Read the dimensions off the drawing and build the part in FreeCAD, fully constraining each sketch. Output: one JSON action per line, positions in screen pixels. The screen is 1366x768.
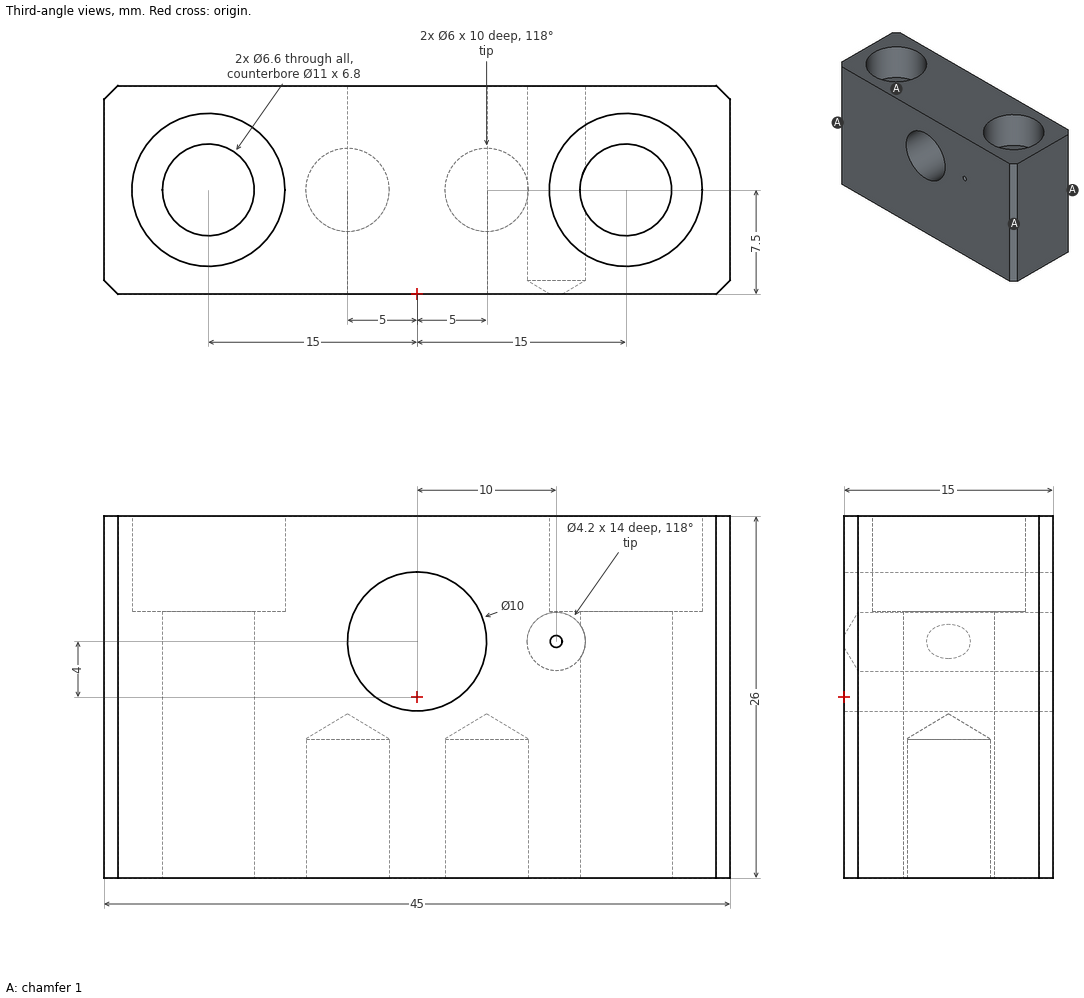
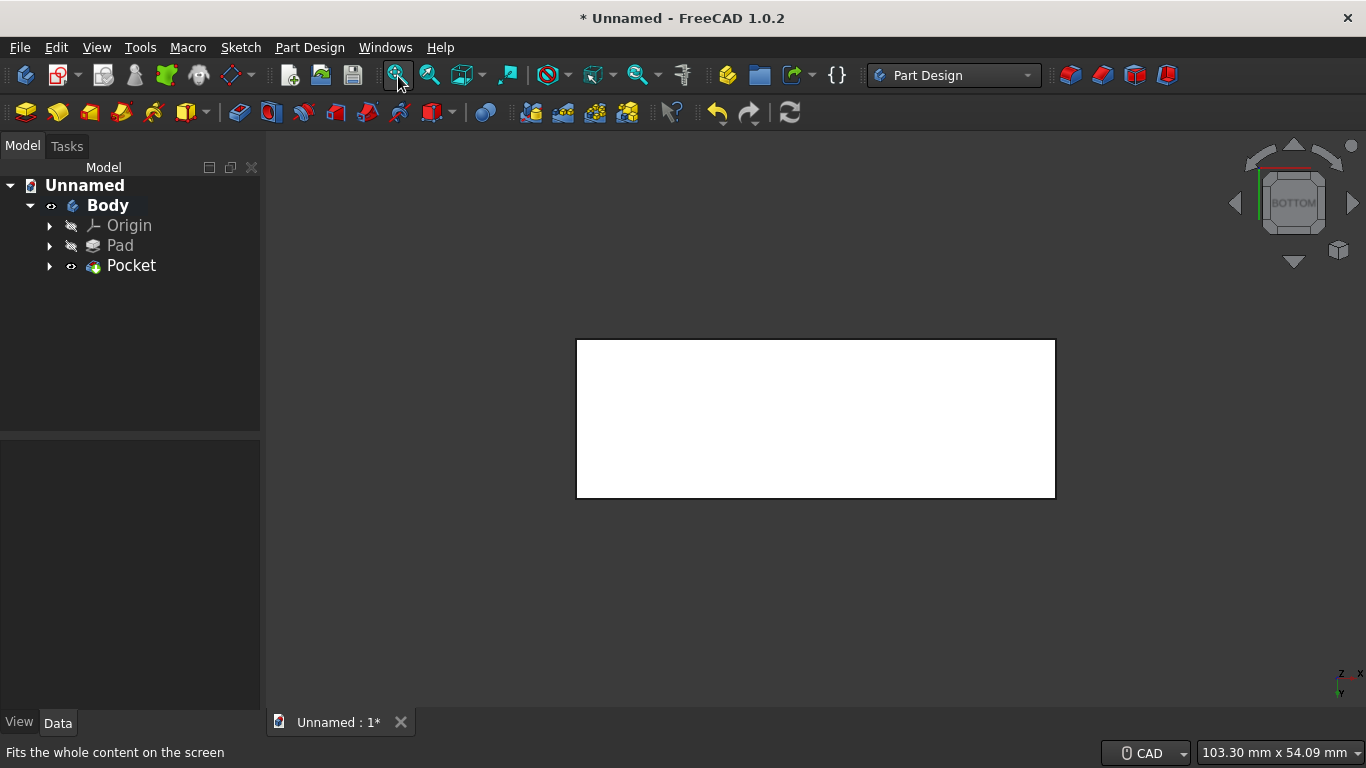
{"action": "left_click", "coordinate": [953, 418]}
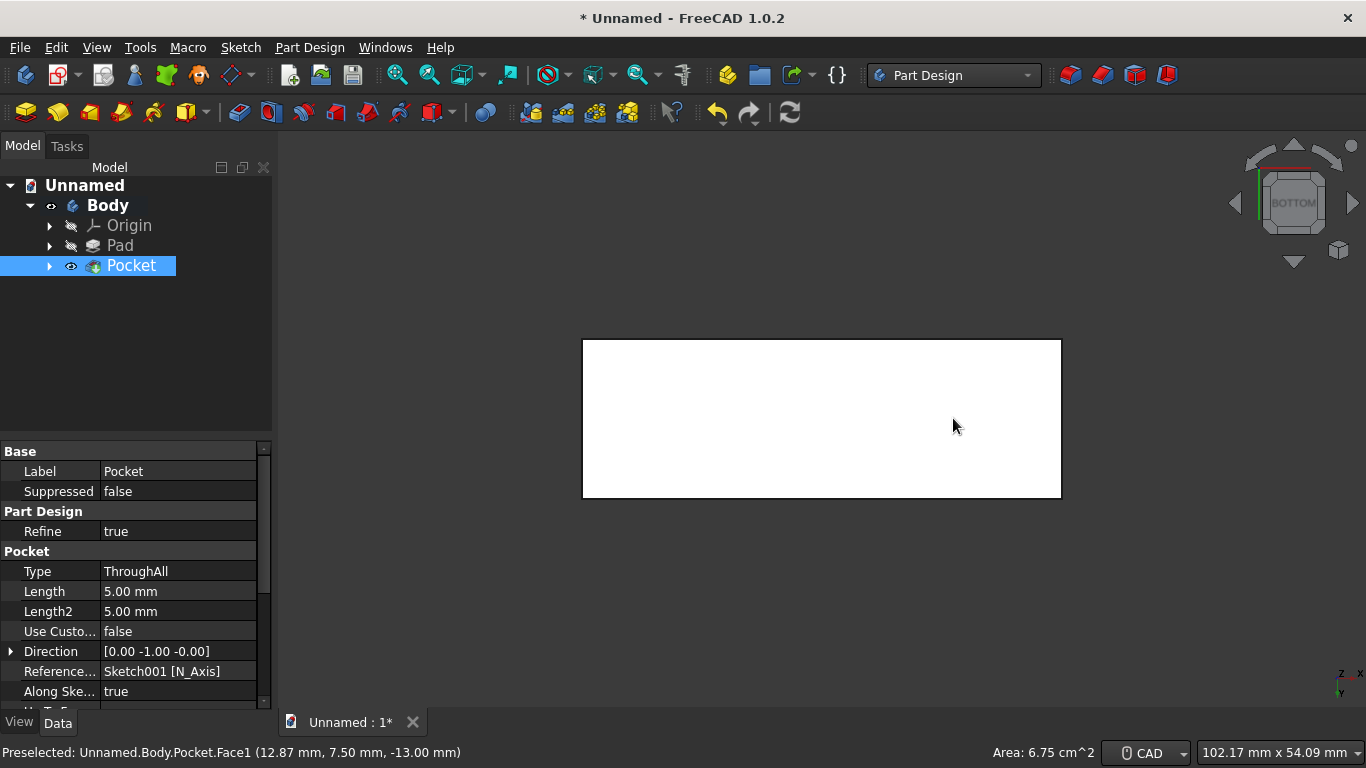
{"action": "left_click", "coordinate": [58, 76]}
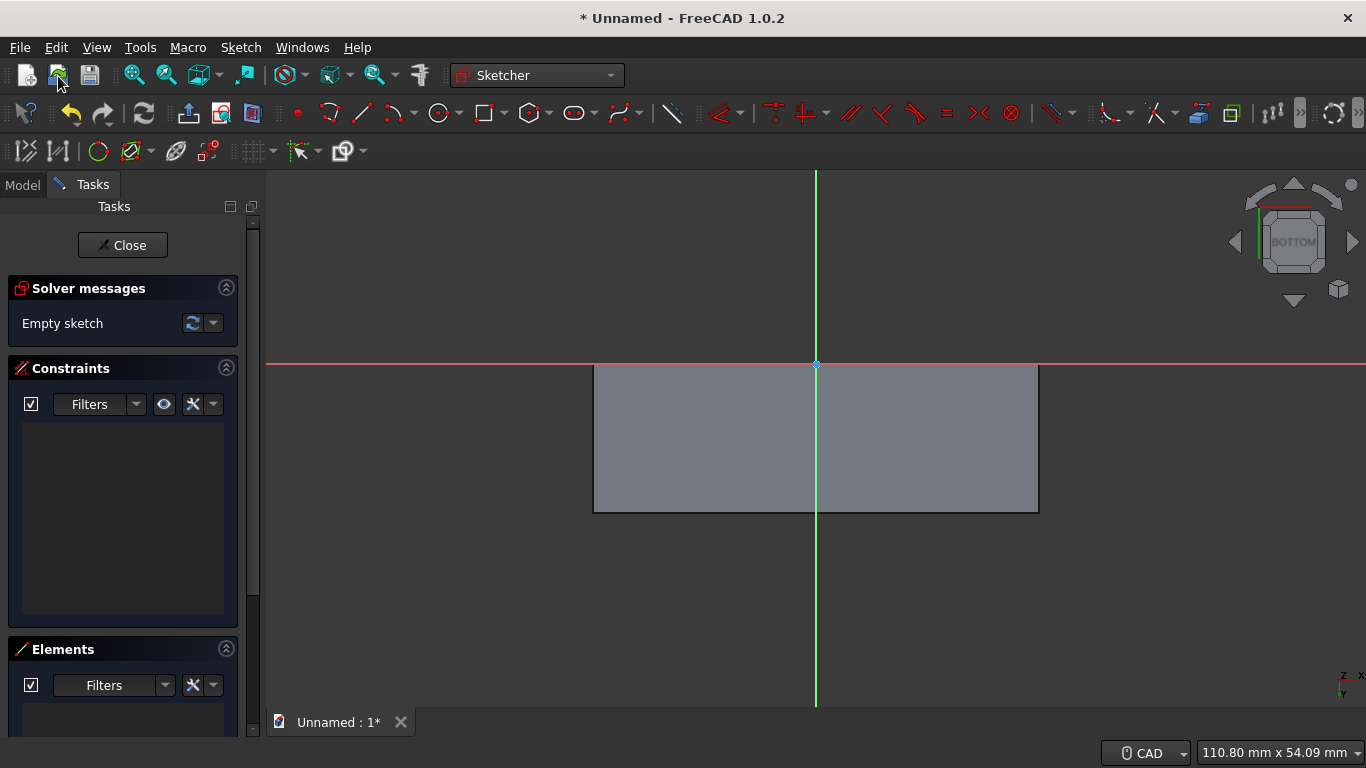
{"action": "scroll", "coordinate": [846, 407], "scroll_direction": "up", "scroll_amount": 6}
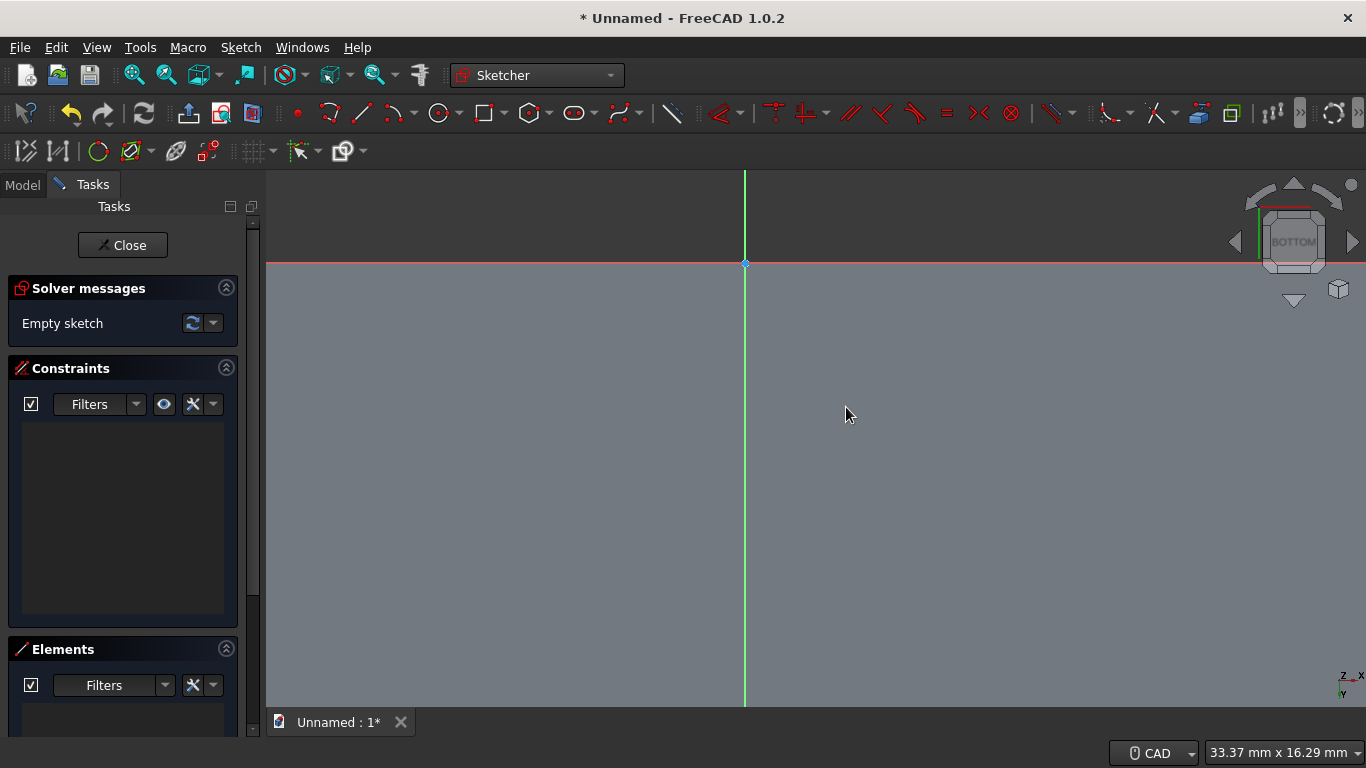
{"action": "left_click", "coordinate": [440, 114]}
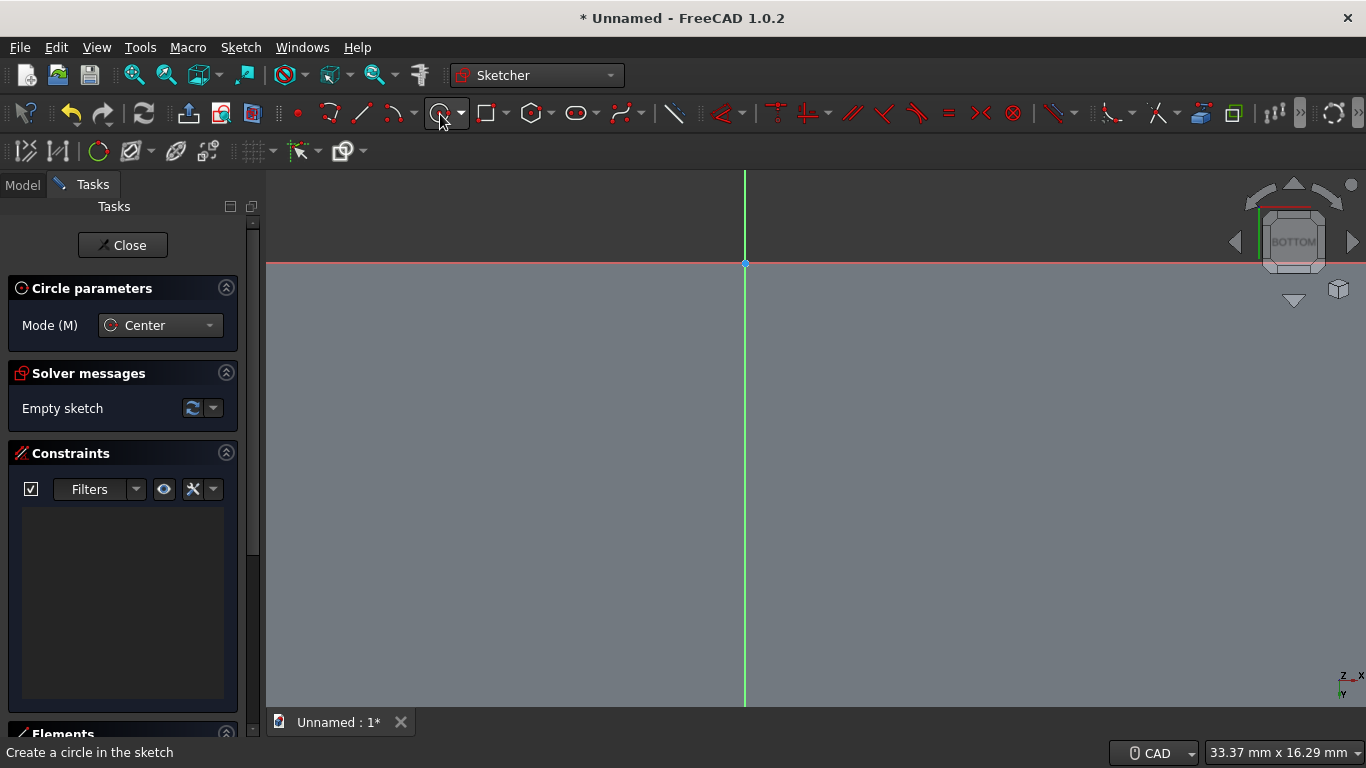
{"action": "left_click", "coordinate": [910, 511]}
{"action": "left_click", "coordinate": [980, 441]}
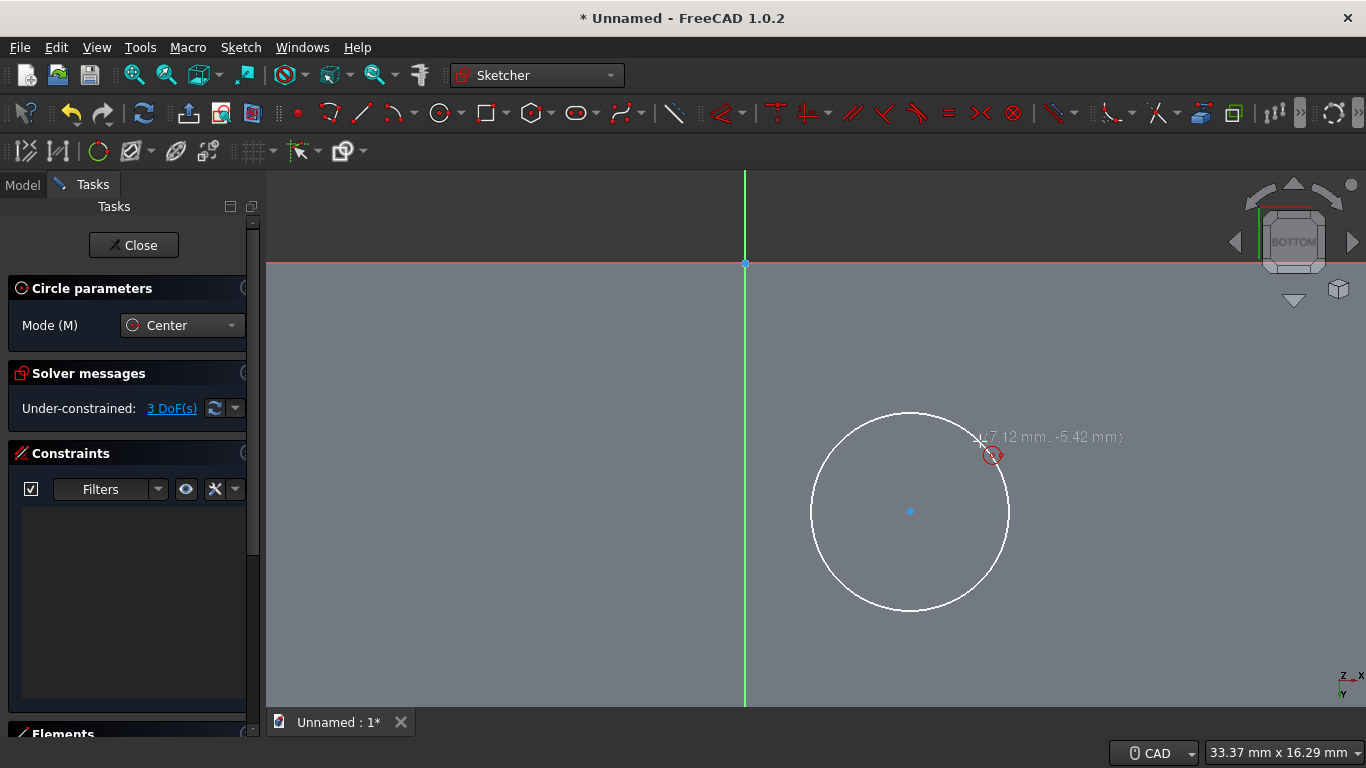
{"action": "left_click", "coordinate": [580, 511]}
{"action": "left_click", "coordinate": [650, 441]}
{"action": "key", "text": "Escape"}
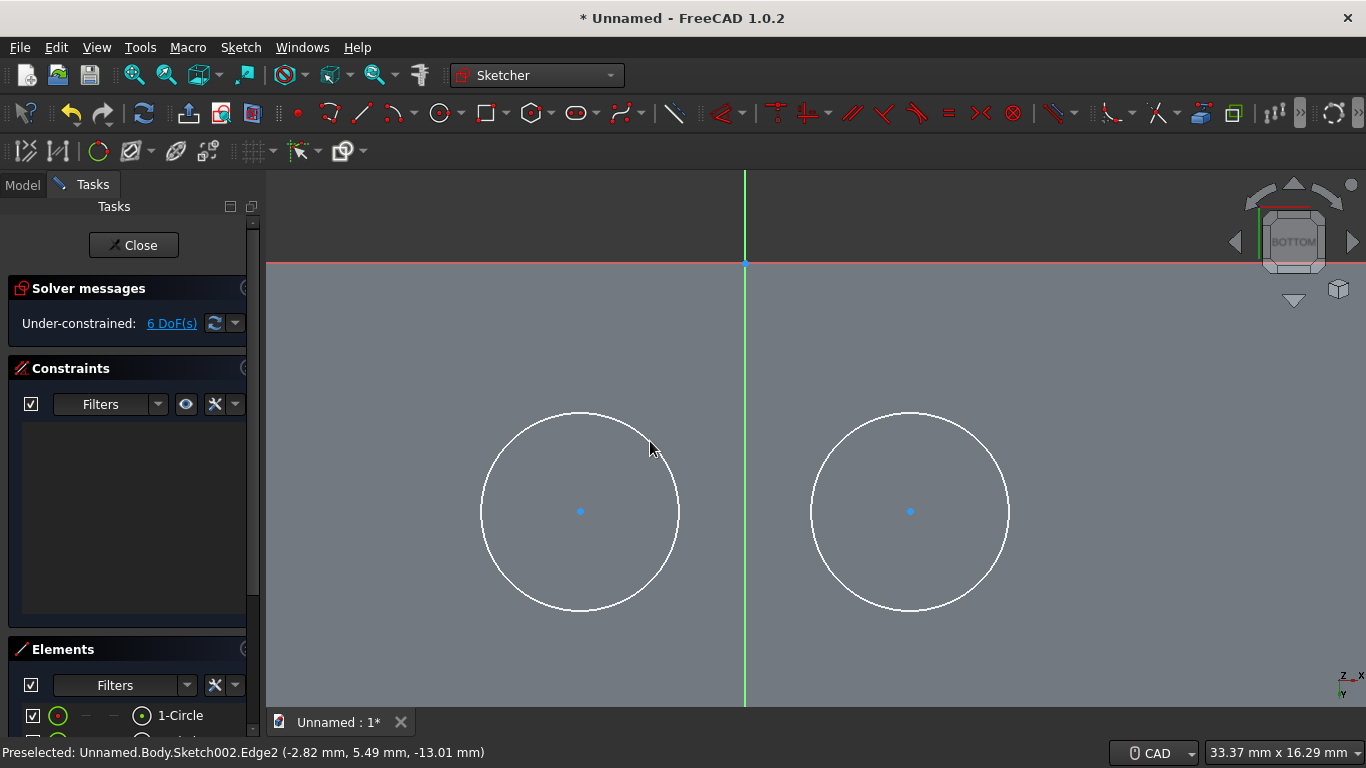
{"action": "left_click", "coordinate": [980, 442]}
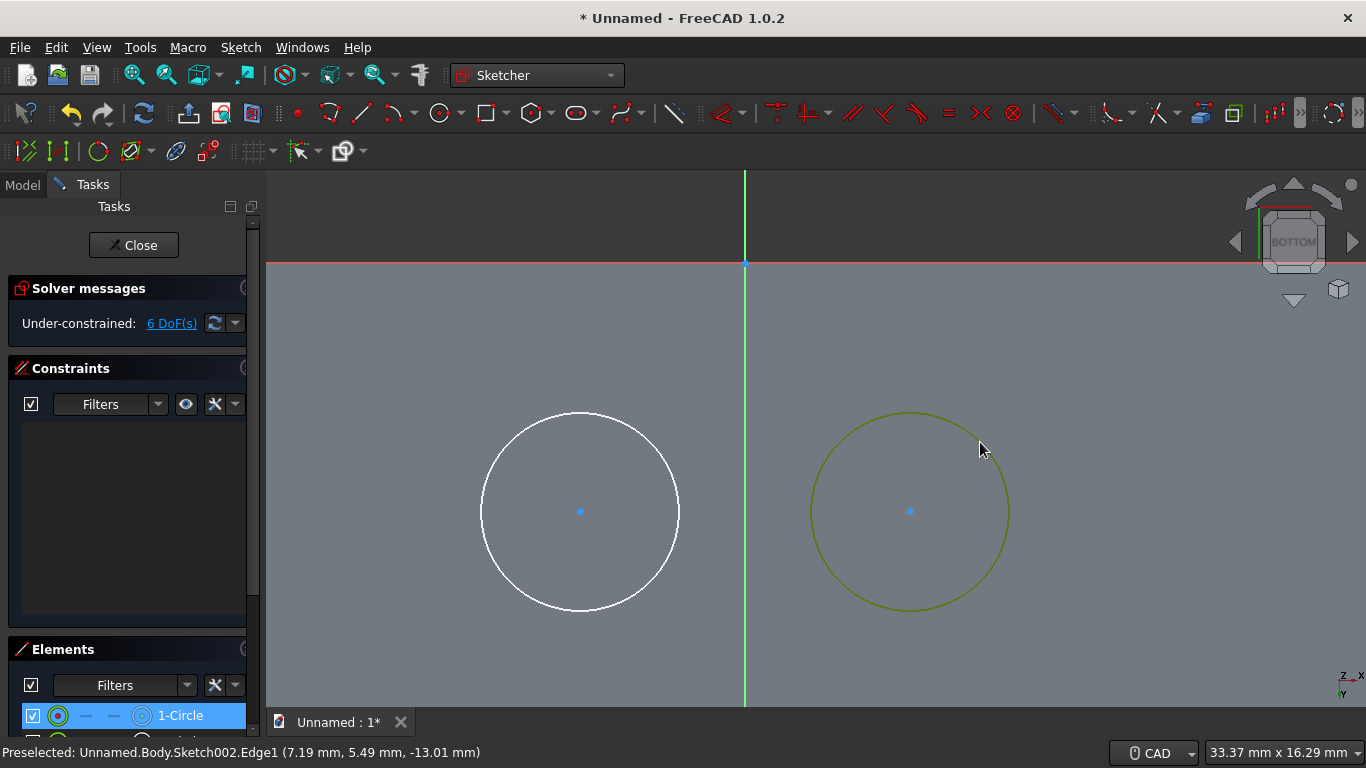
{"action": "left_click", "coordinate": [650, 442]}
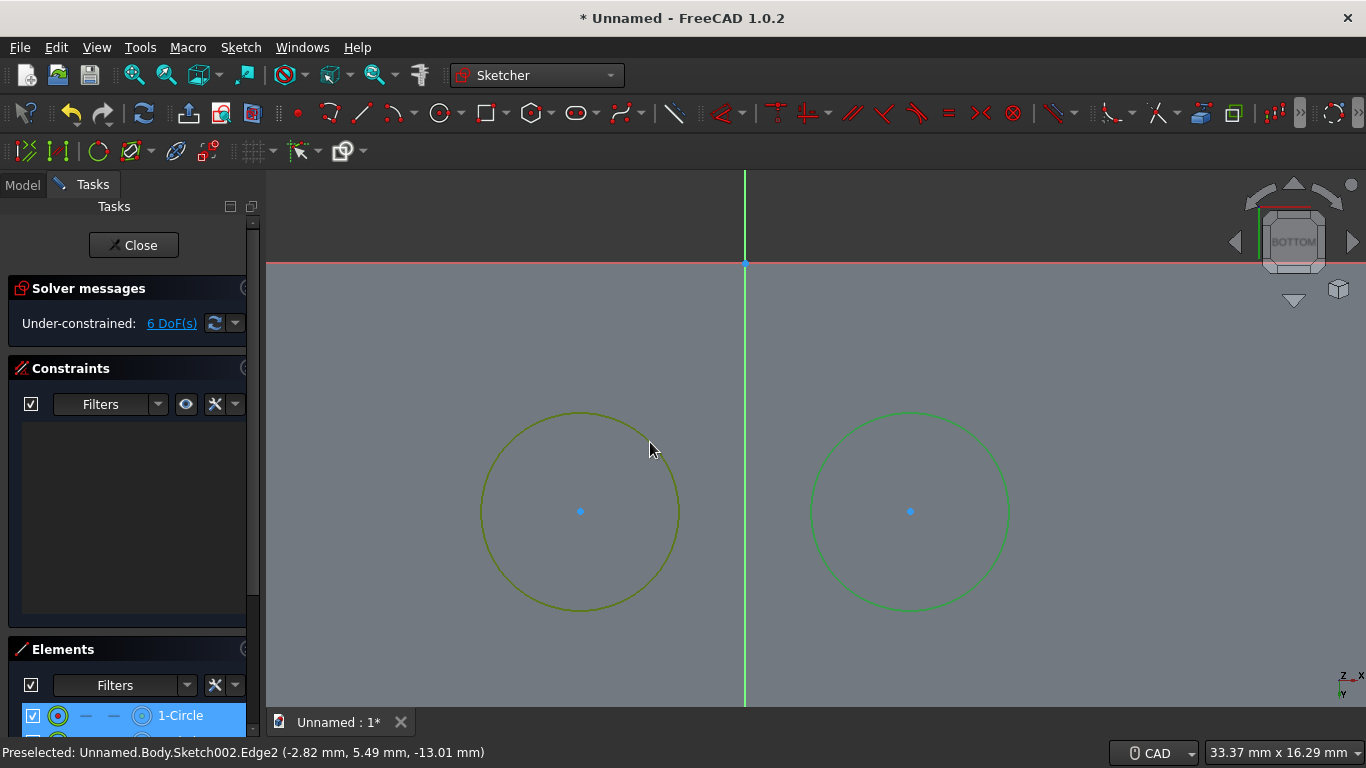
{"action": "left_click", "coordinate": [950, 114]}